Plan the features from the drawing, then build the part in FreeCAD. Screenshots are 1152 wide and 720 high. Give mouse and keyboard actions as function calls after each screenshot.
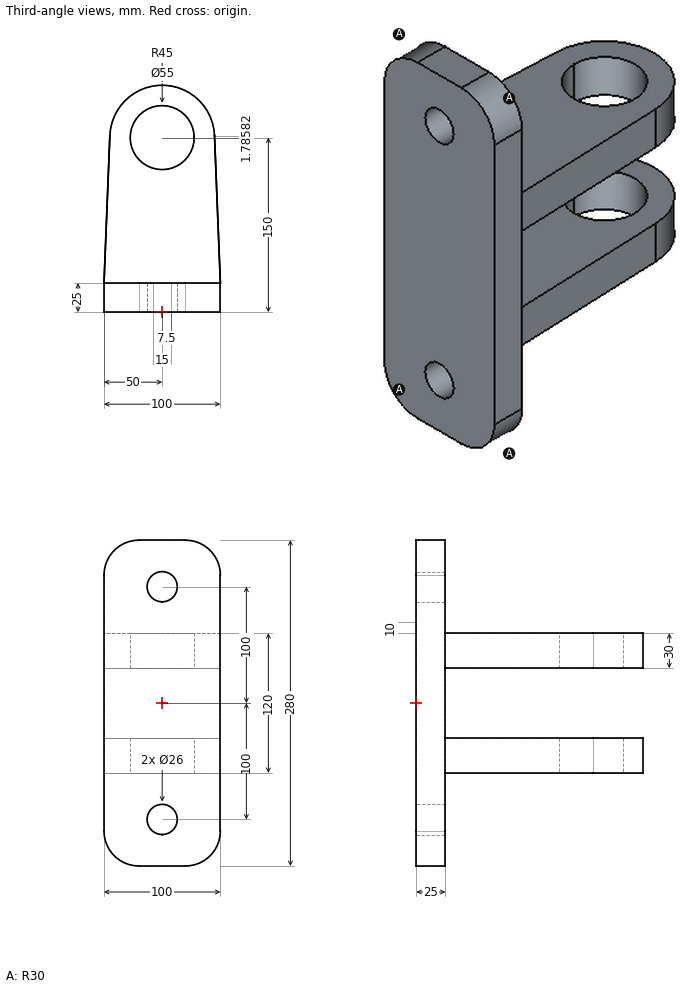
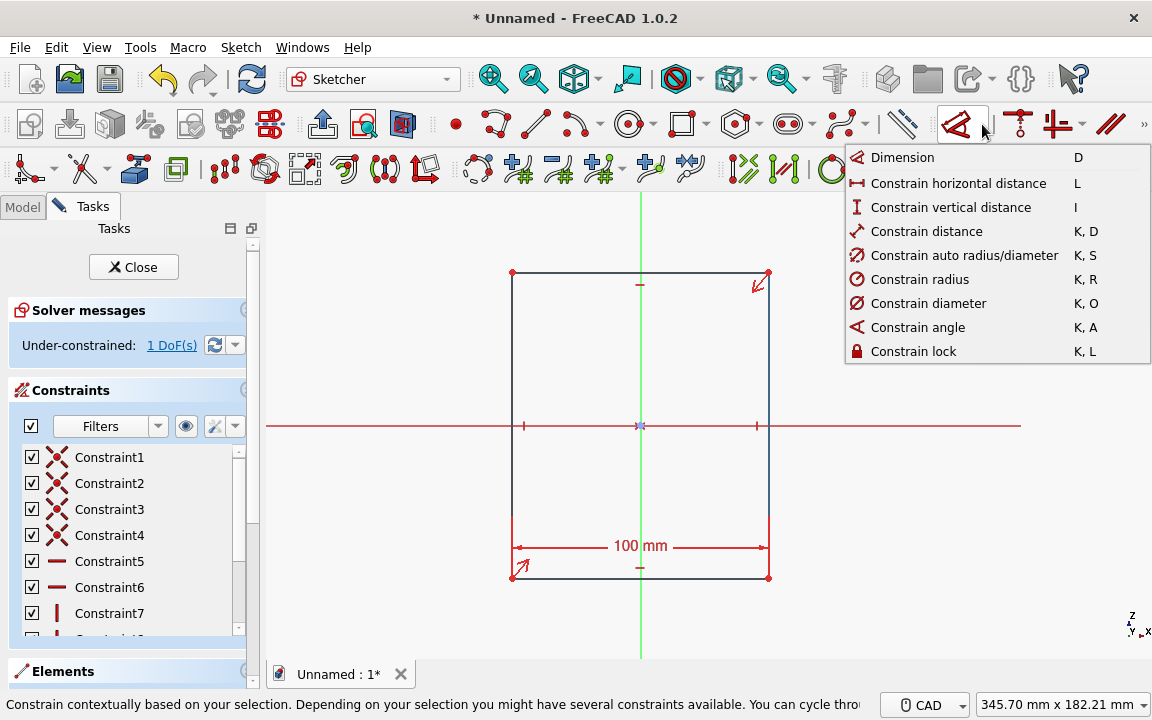
click(998, 207)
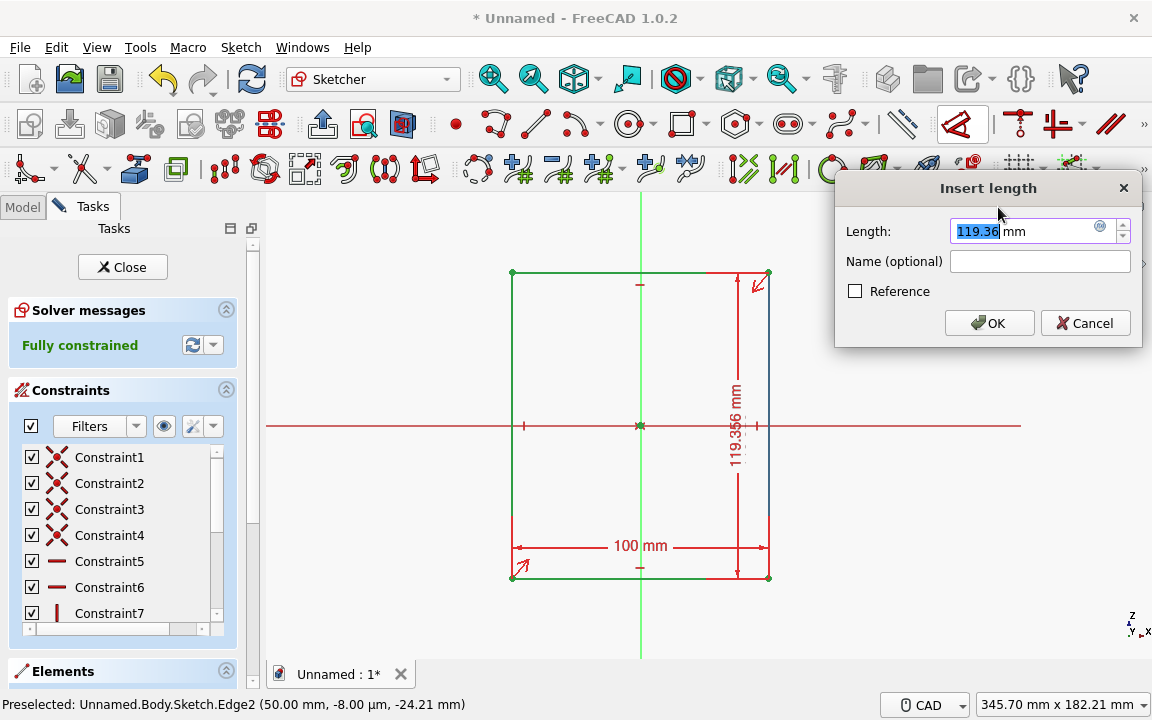
text(120)
key(Return)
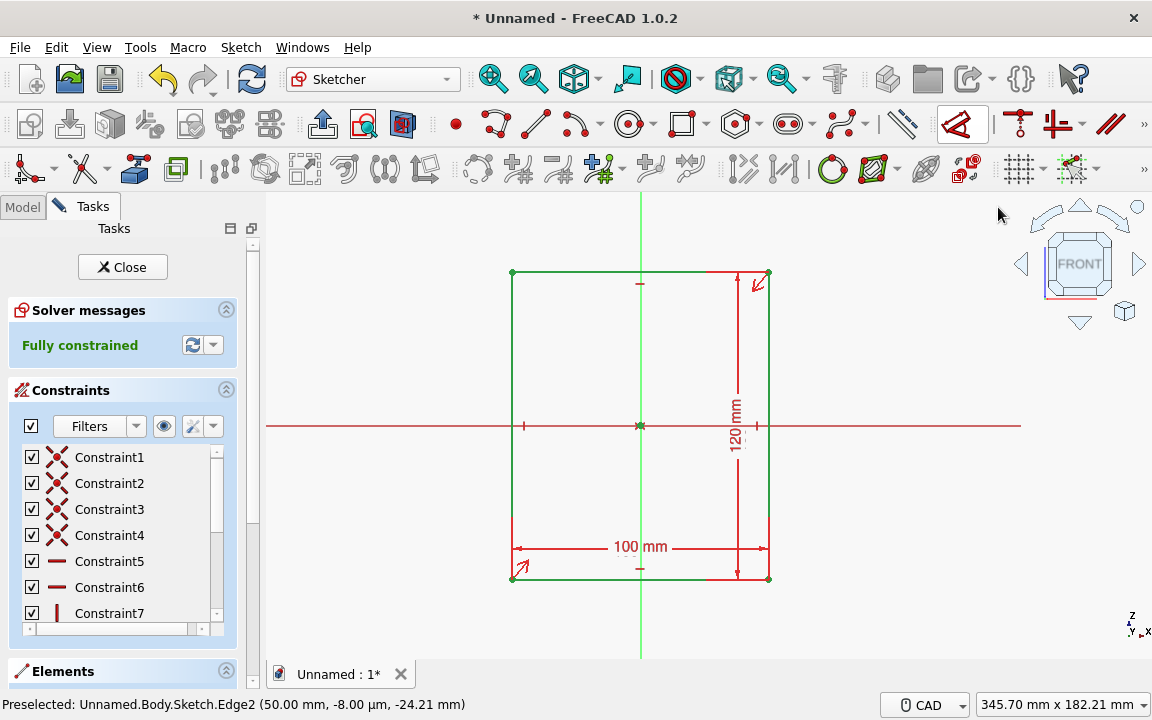
click(123, 267)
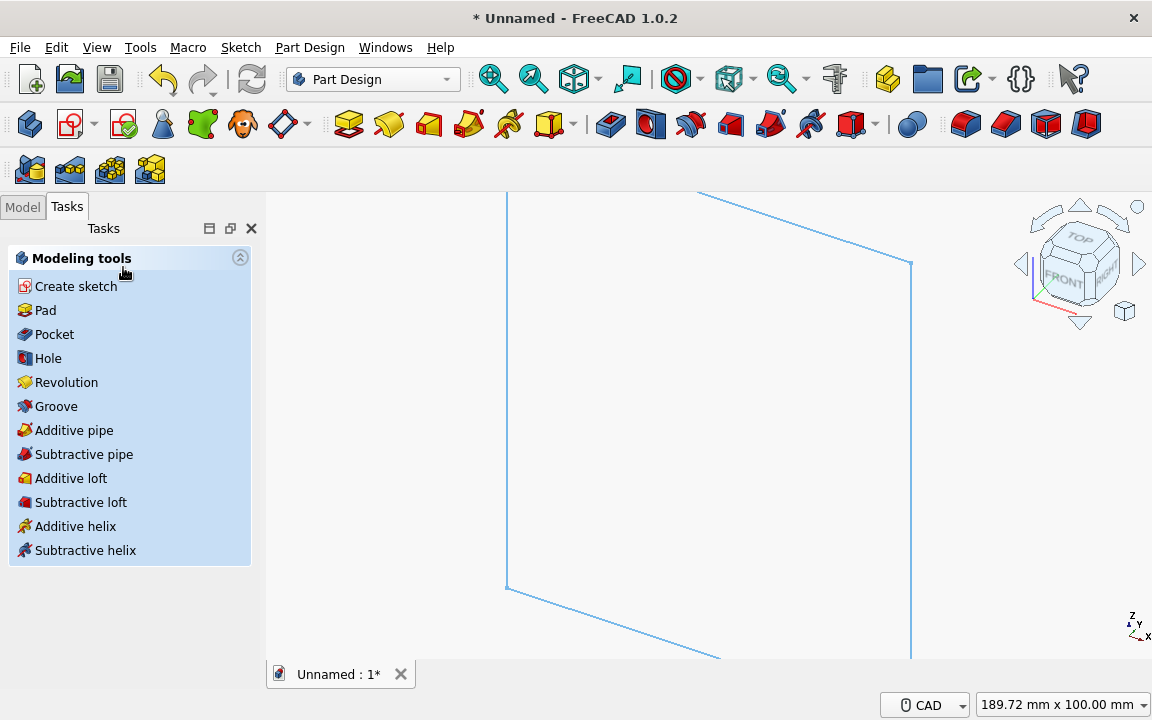
click(350, 124)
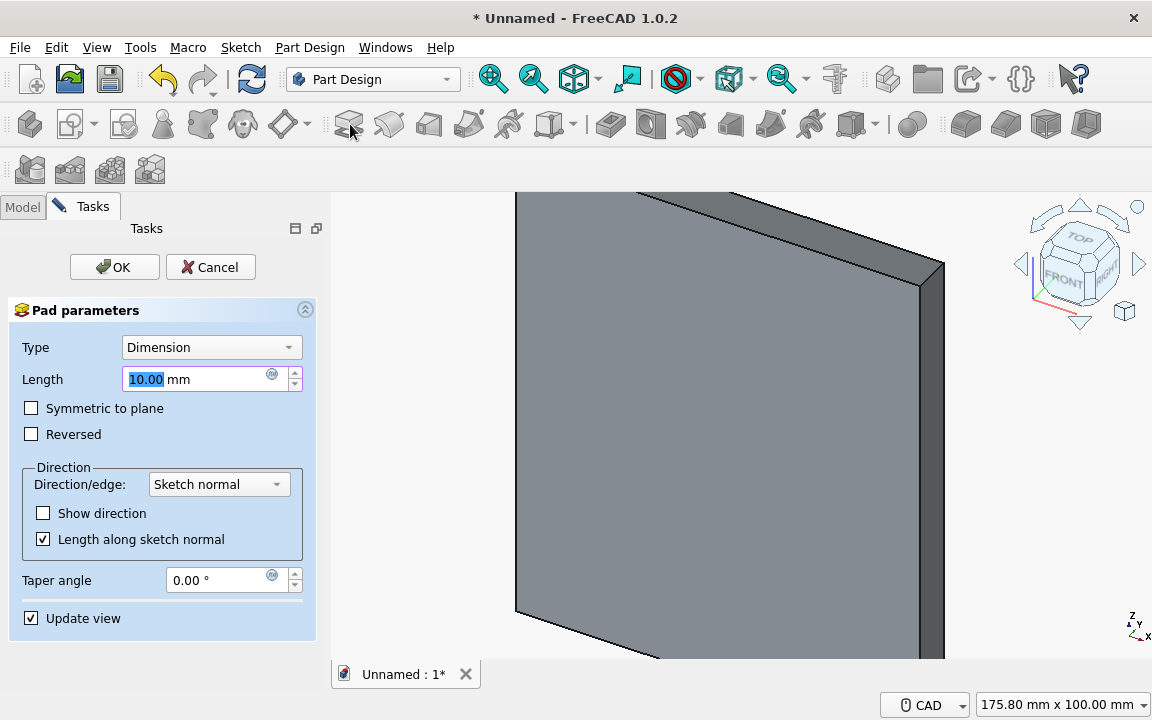
text(25)
key(Tab)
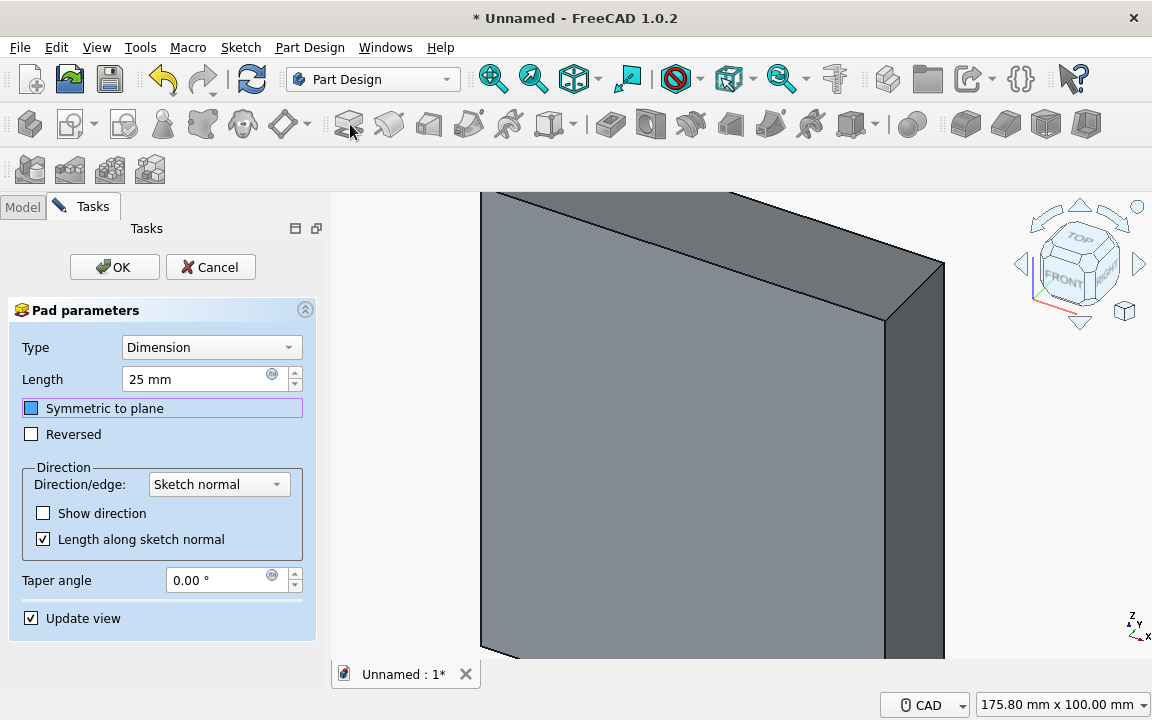
click(30, 434)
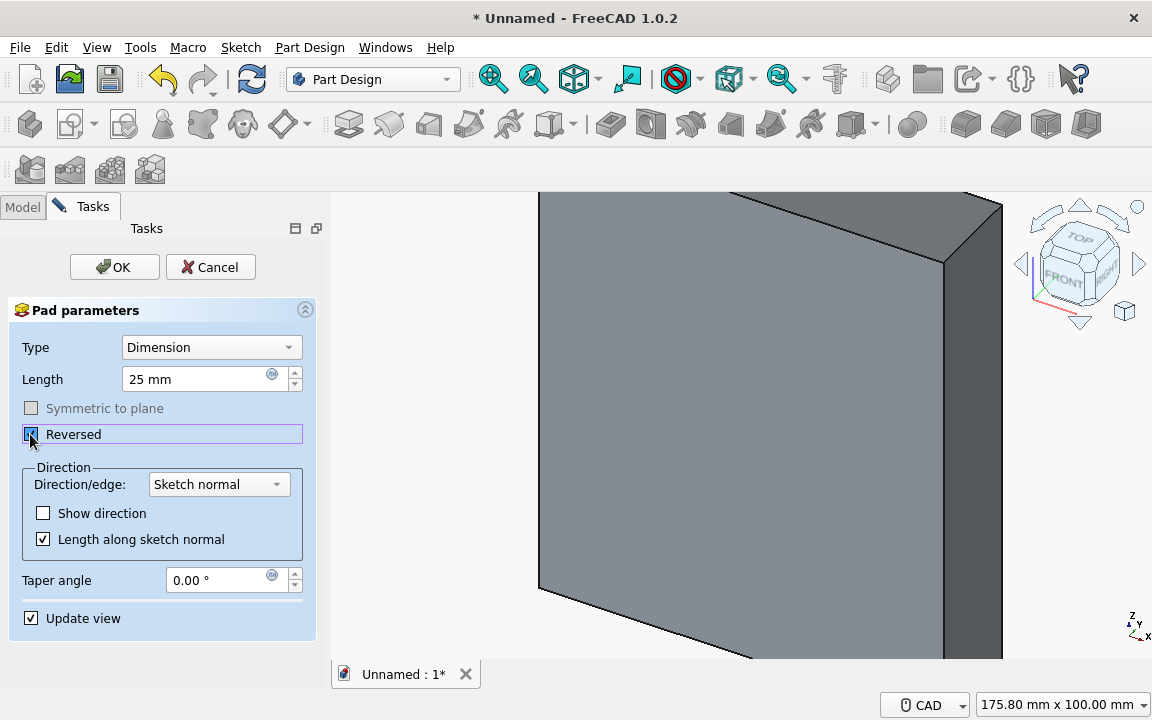
click(115, 267)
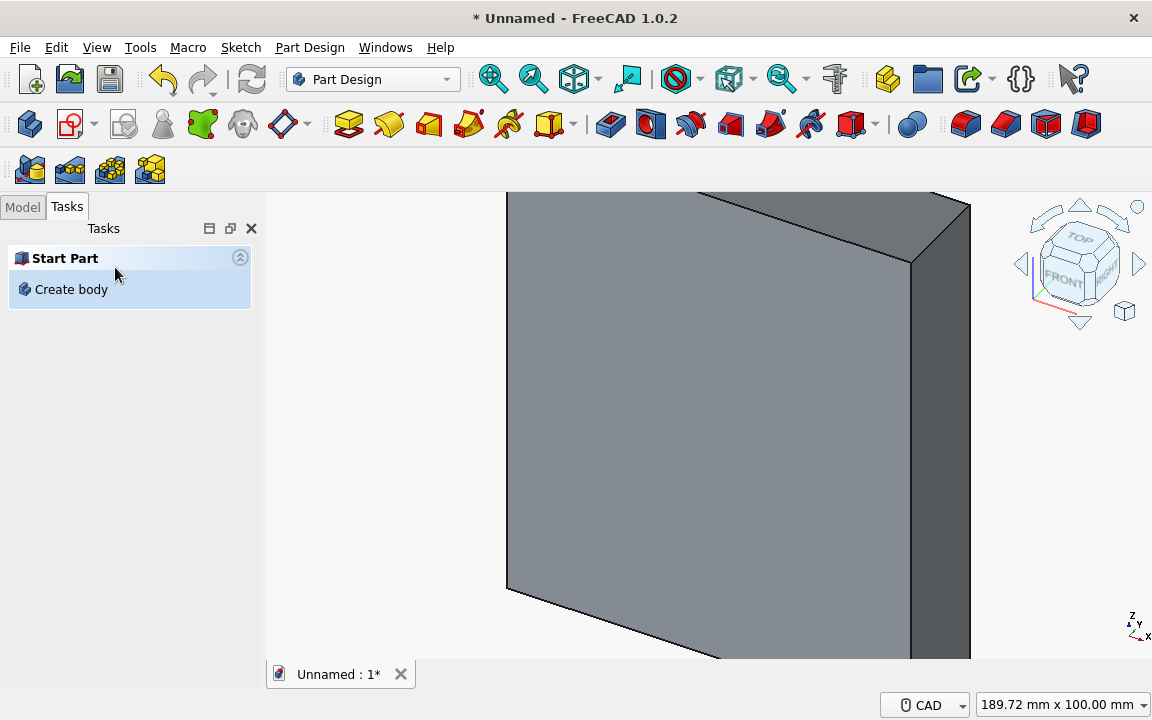
click(494, 80)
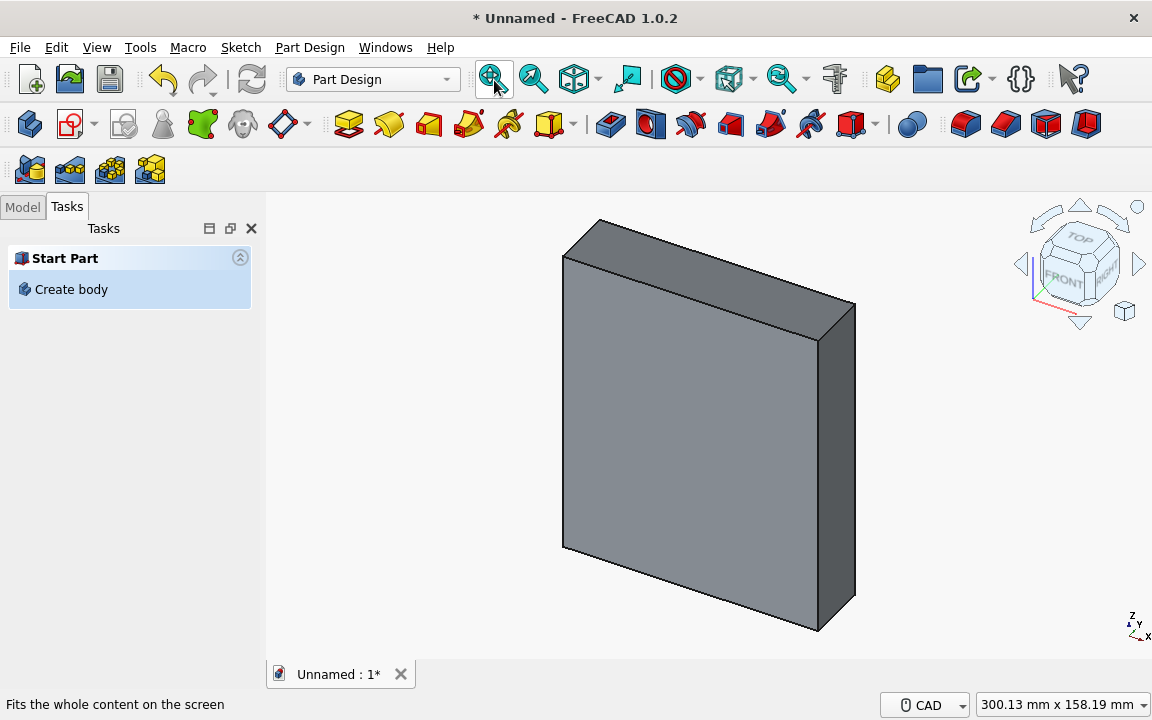
click(782, 304)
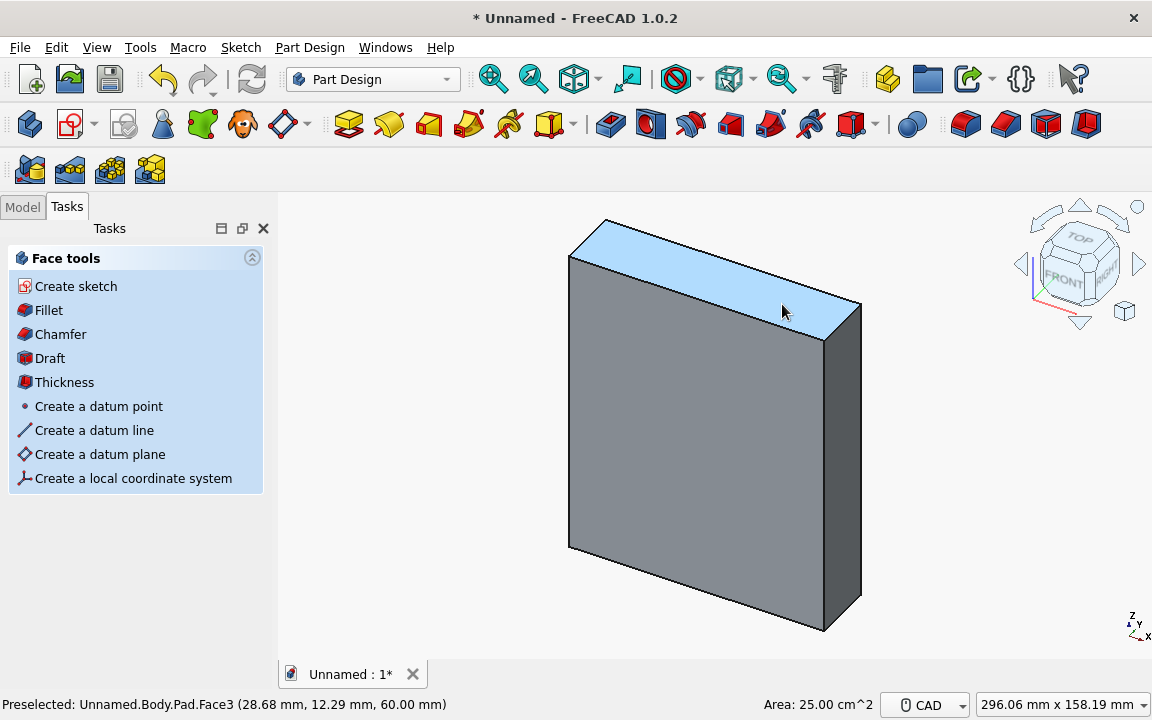
click(70, 124)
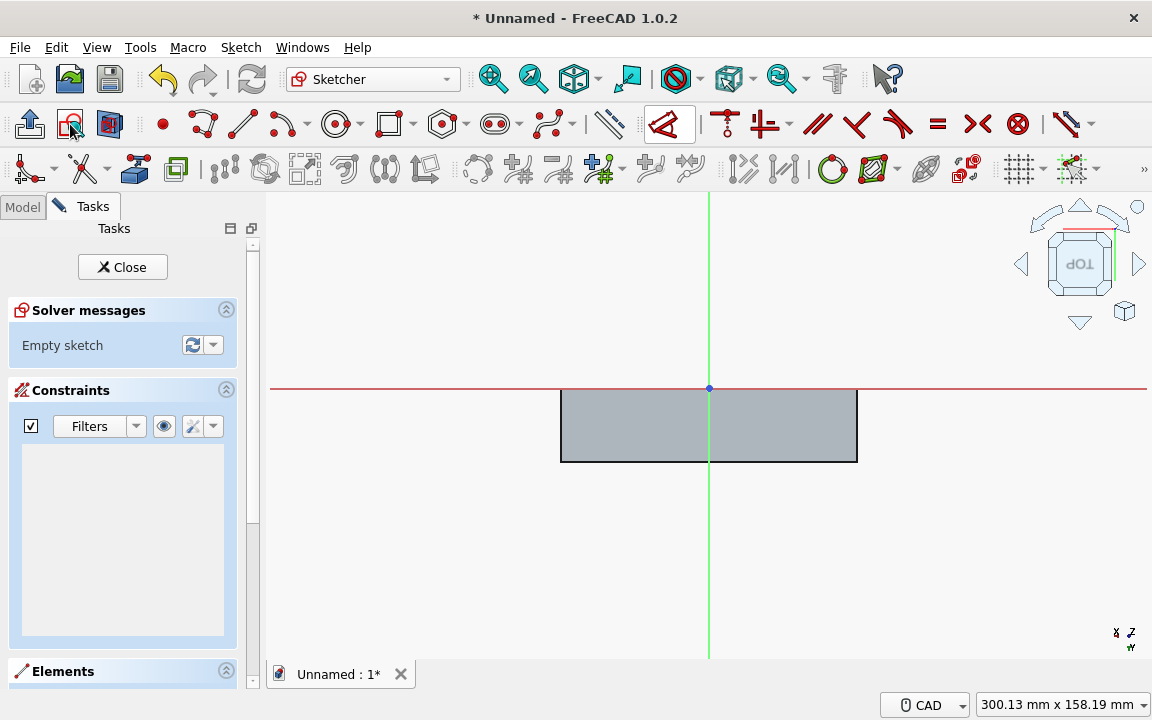
scroll(585, 221, down, 4)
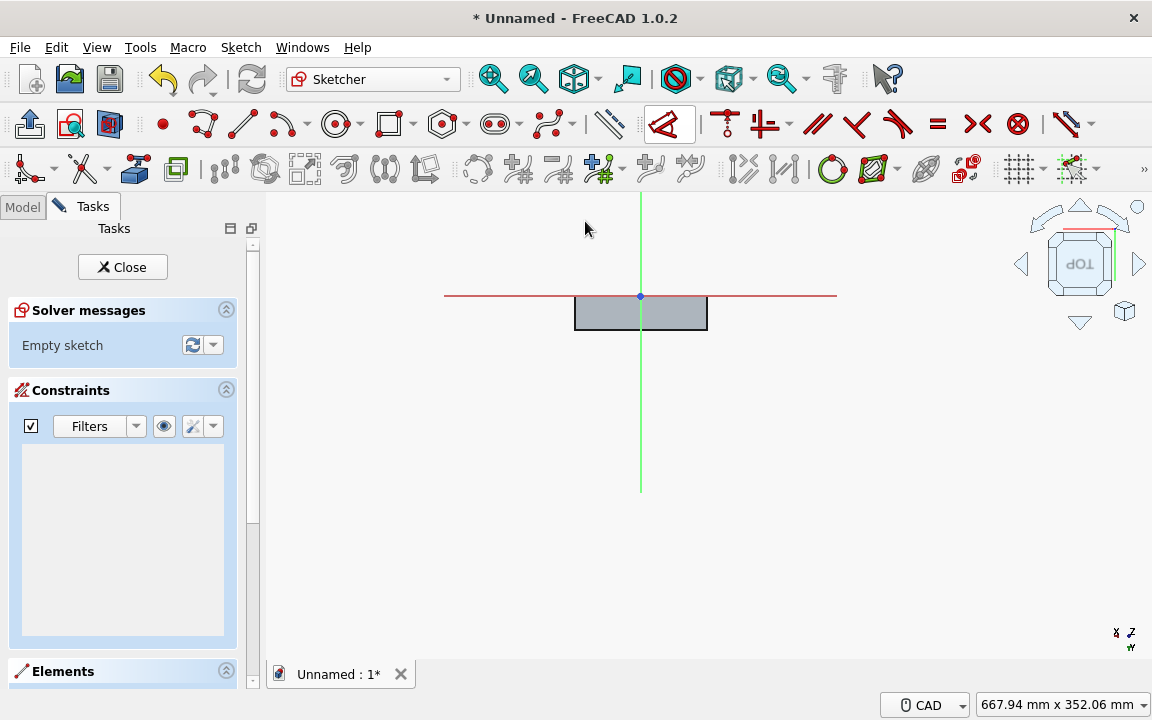
click(204, 124)